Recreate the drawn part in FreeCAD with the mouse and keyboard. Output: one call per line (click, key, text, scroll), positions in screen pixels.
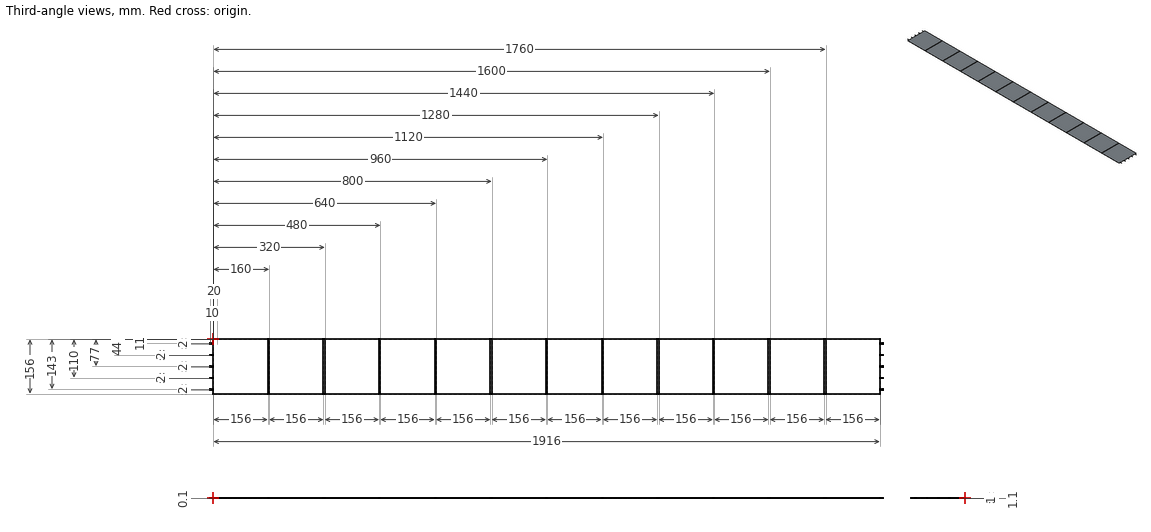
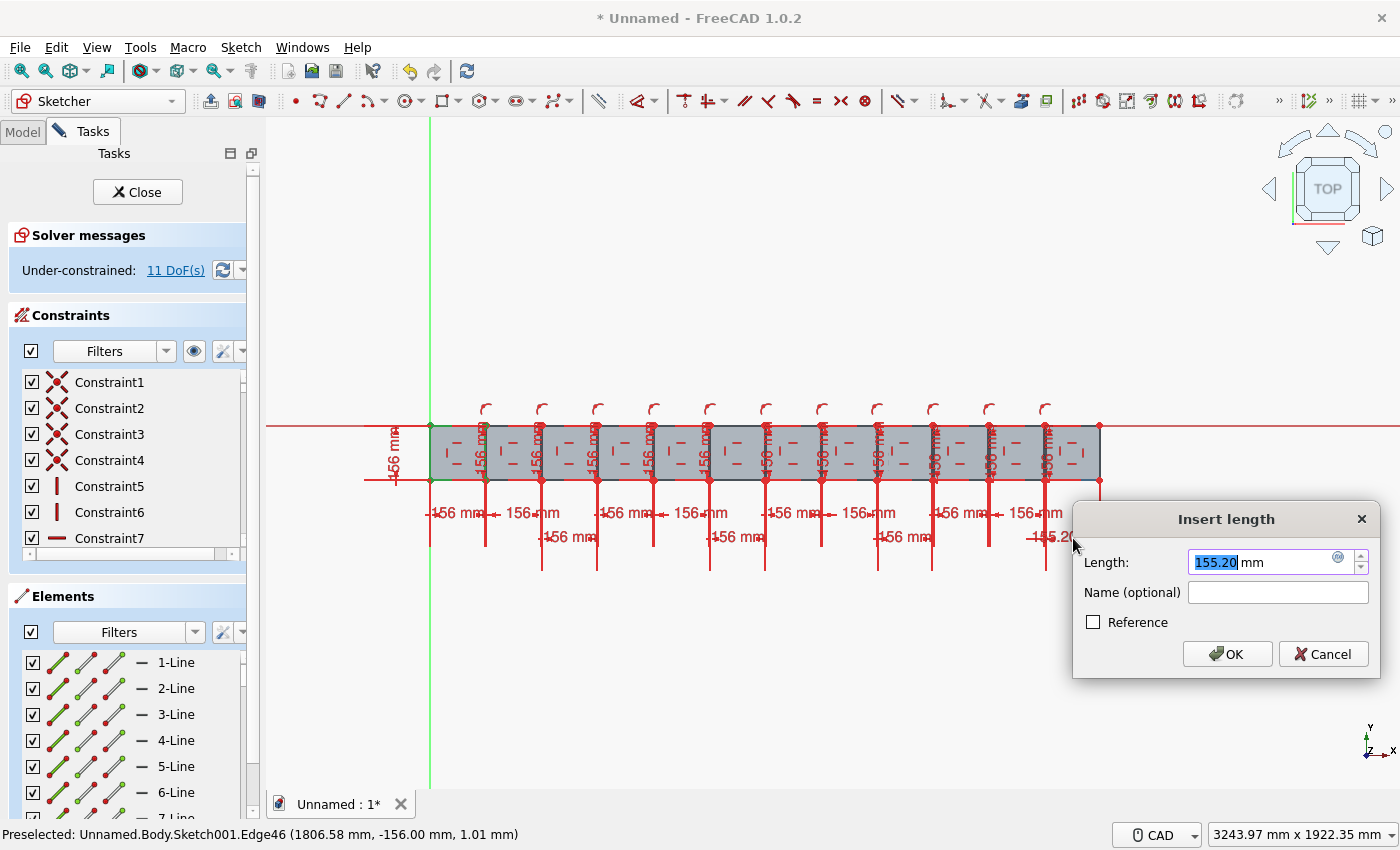
text(156)
key(Return)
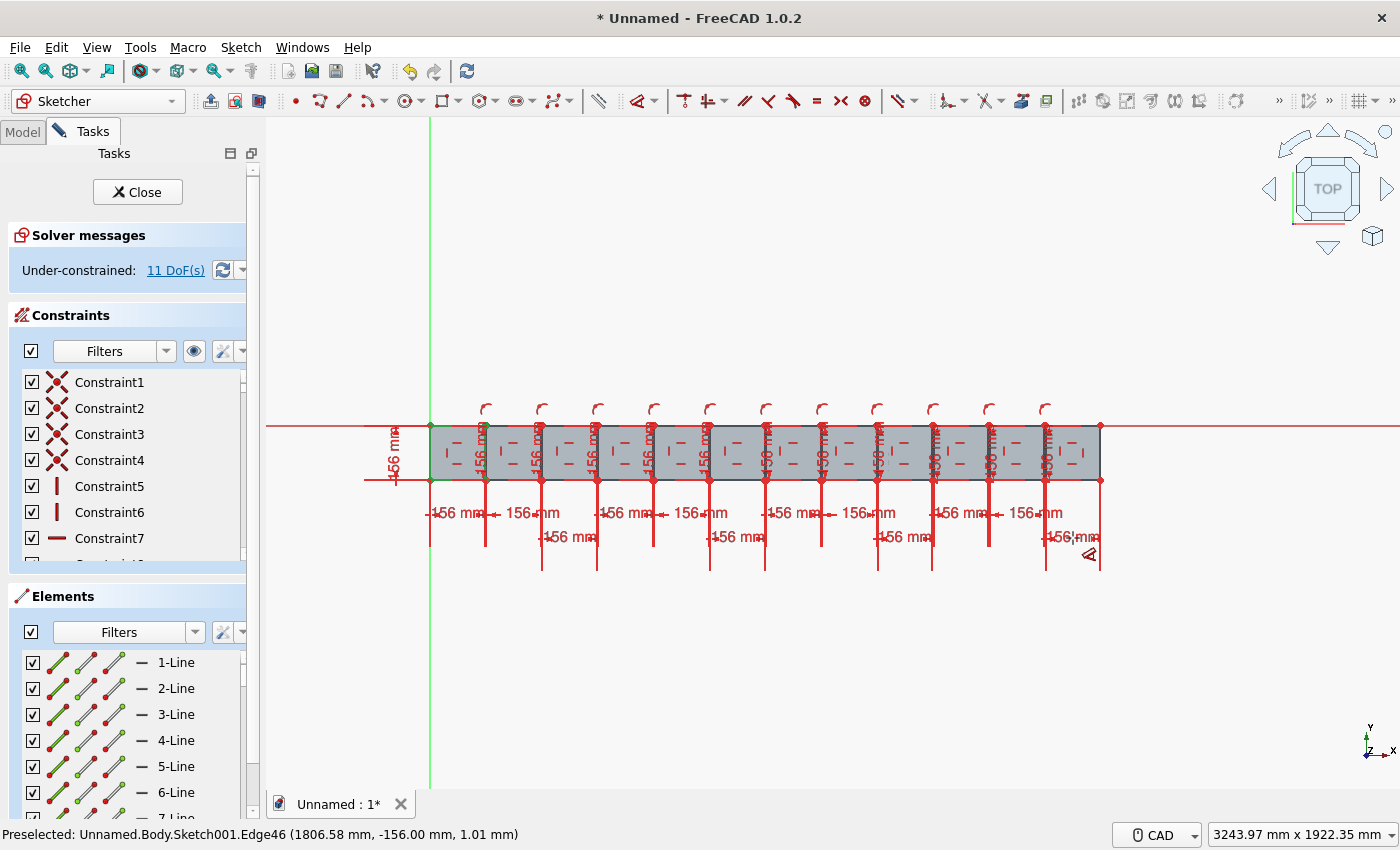
scroll(486, 426, up, 11)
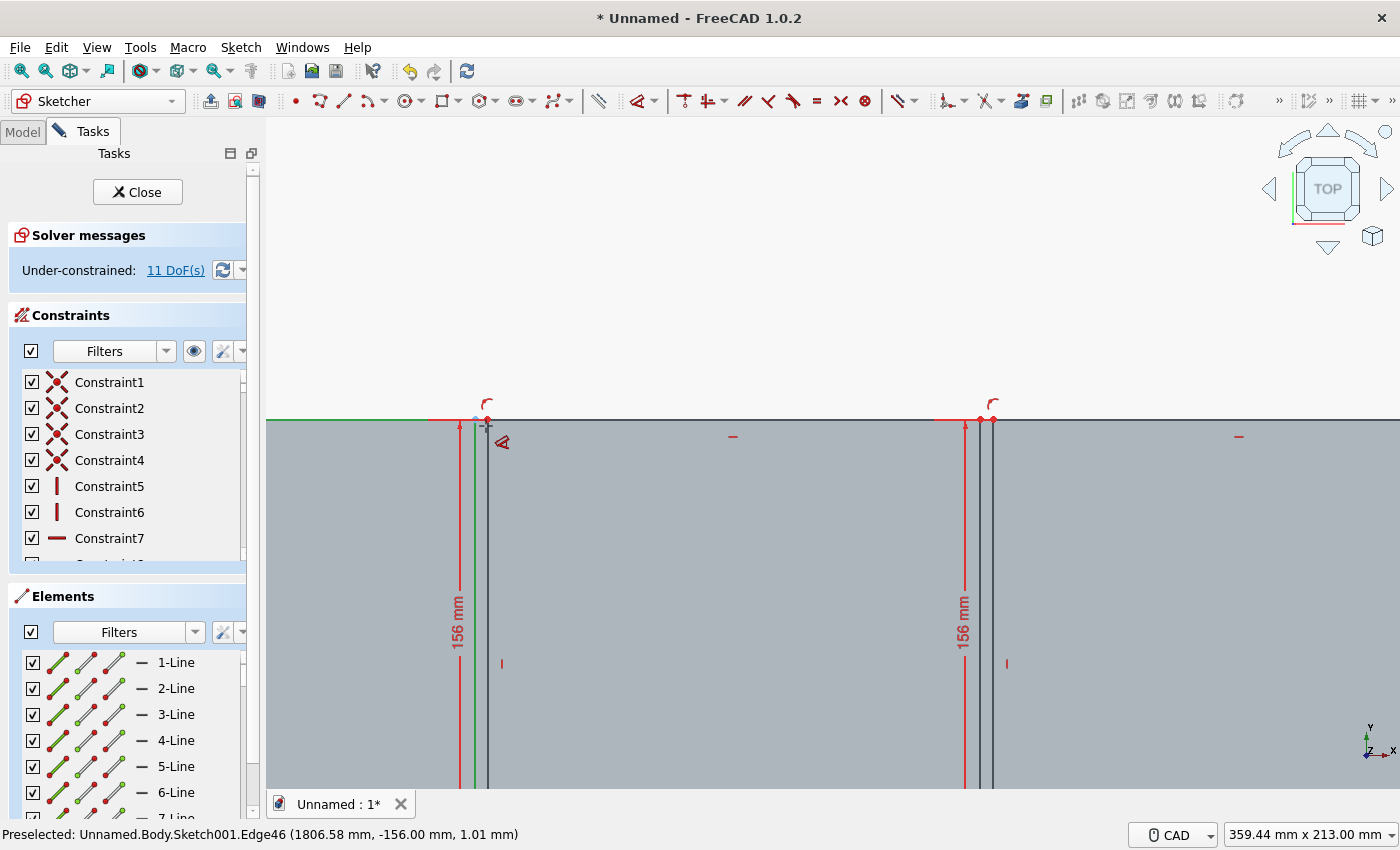
click(488, 420)
click(391, 386)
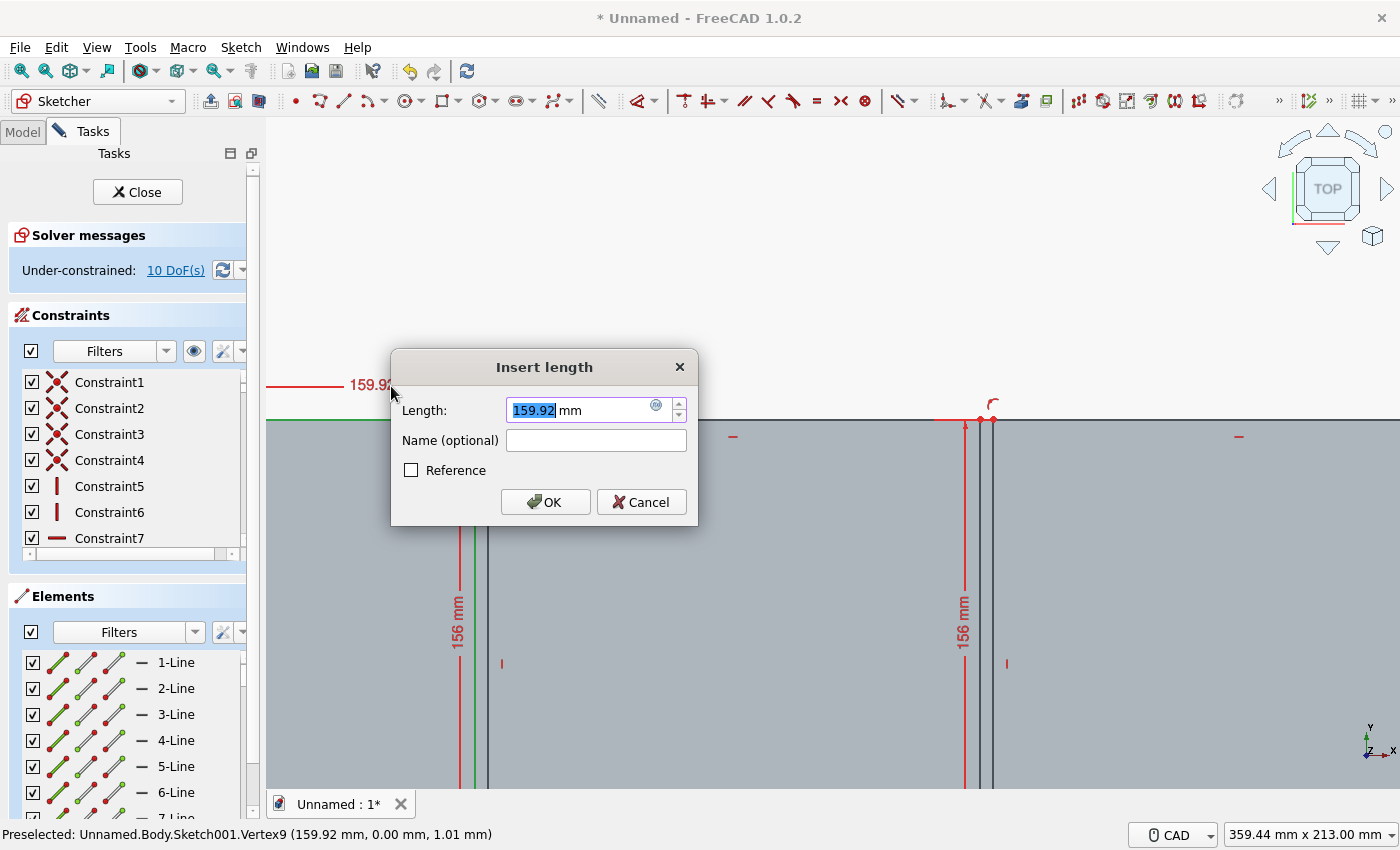
text(160)
key(Return)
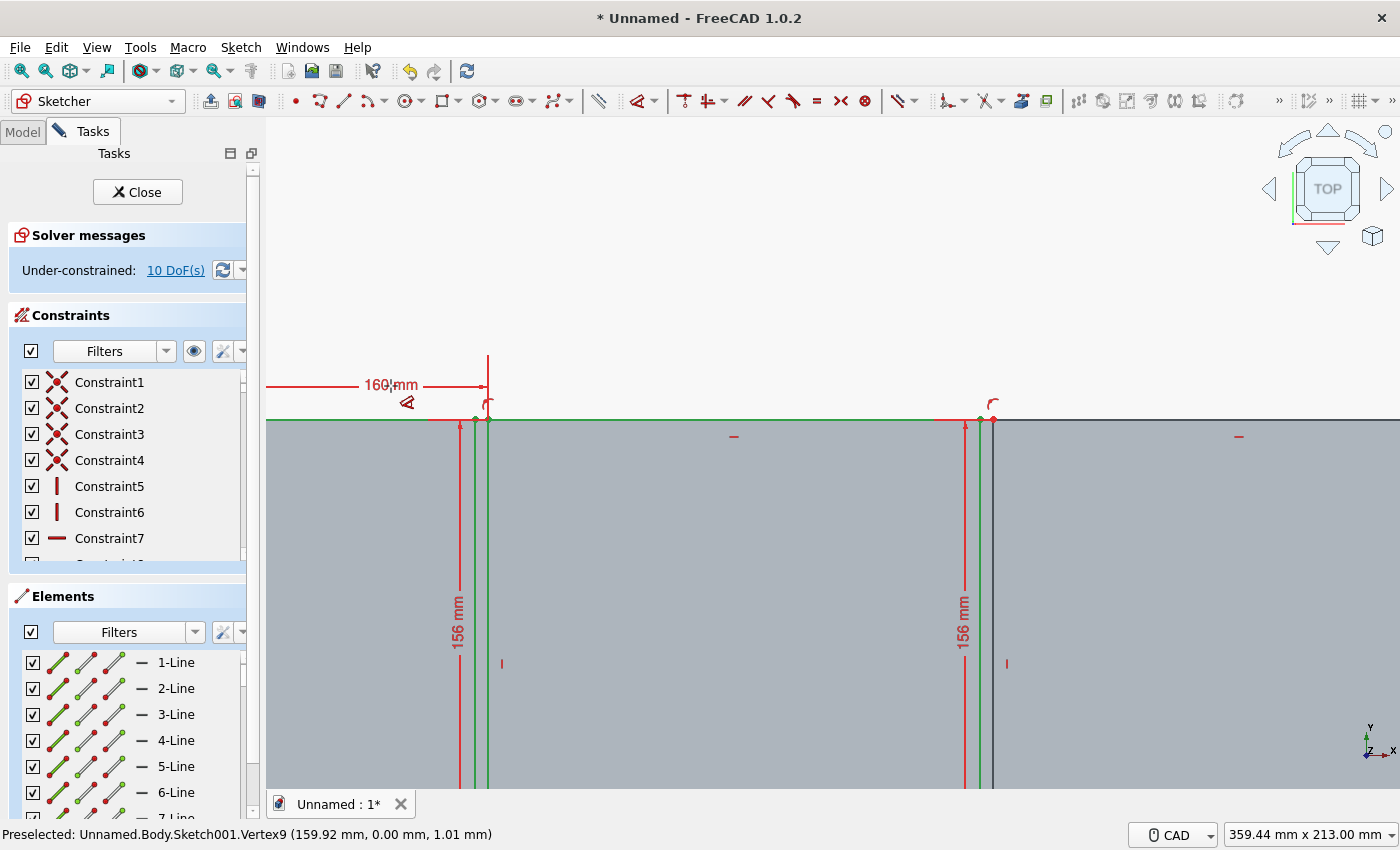
click(993, 420)
click(644, 386)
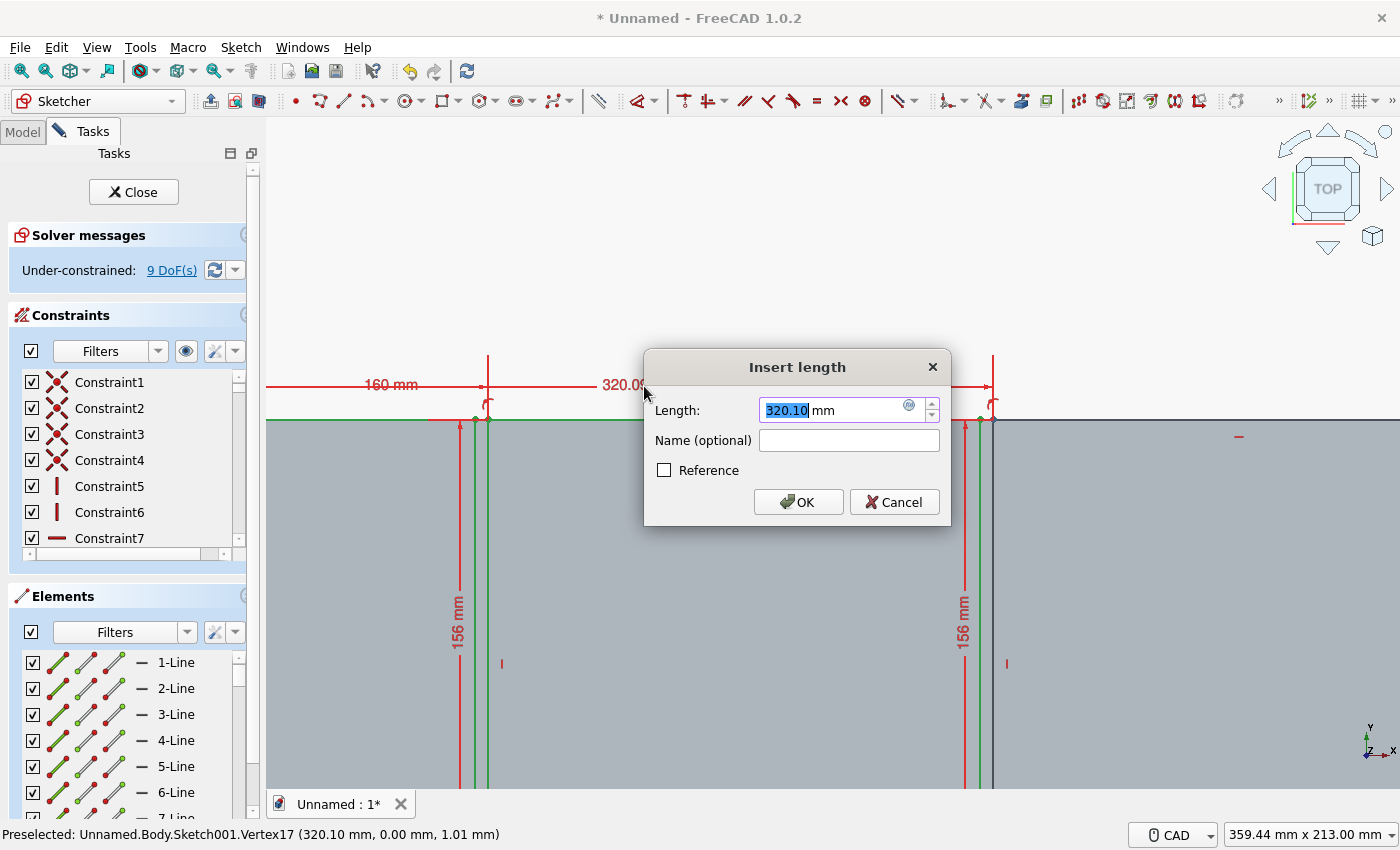
text(320)
key(Return)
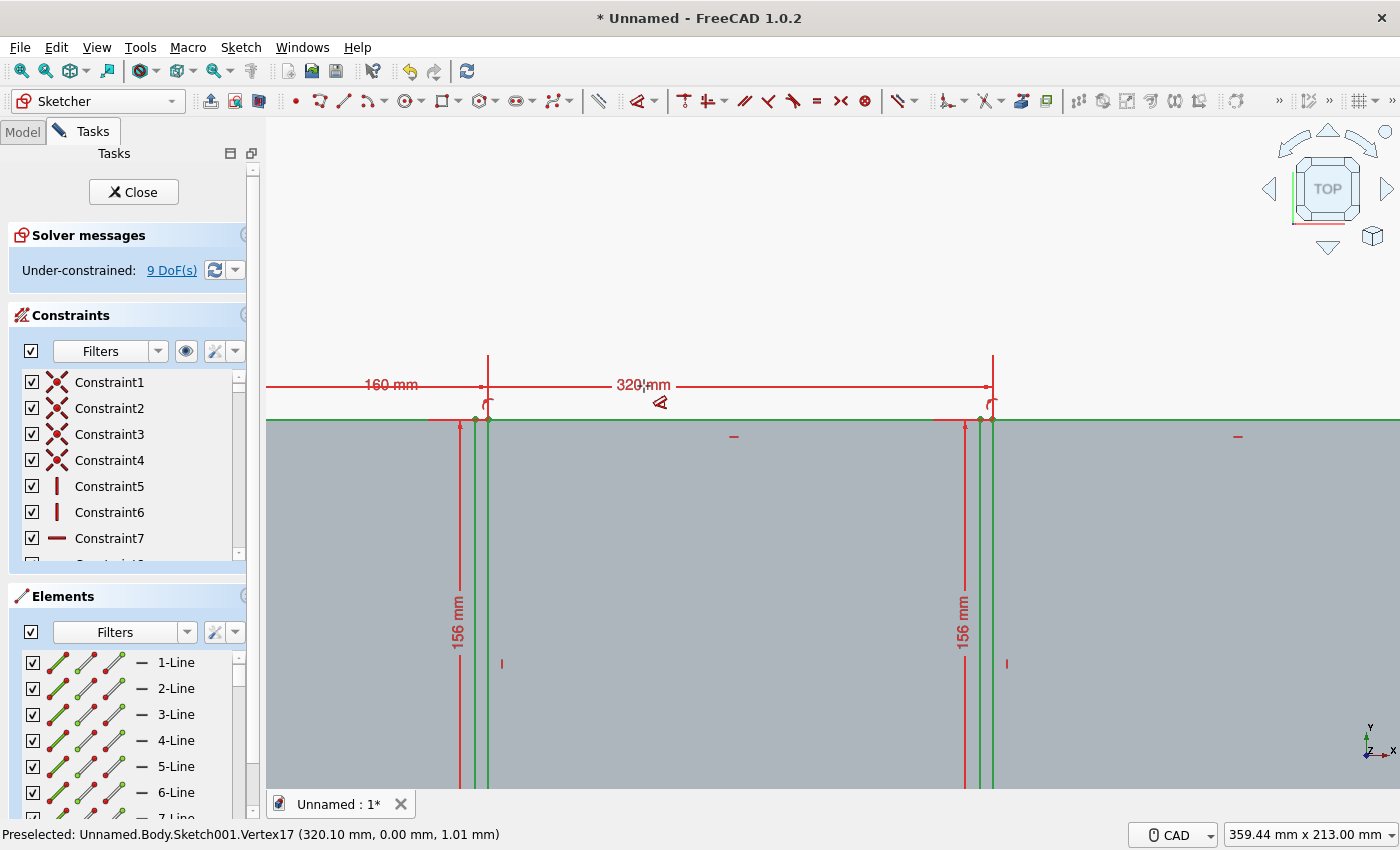
scroll(485, 426, down, 11)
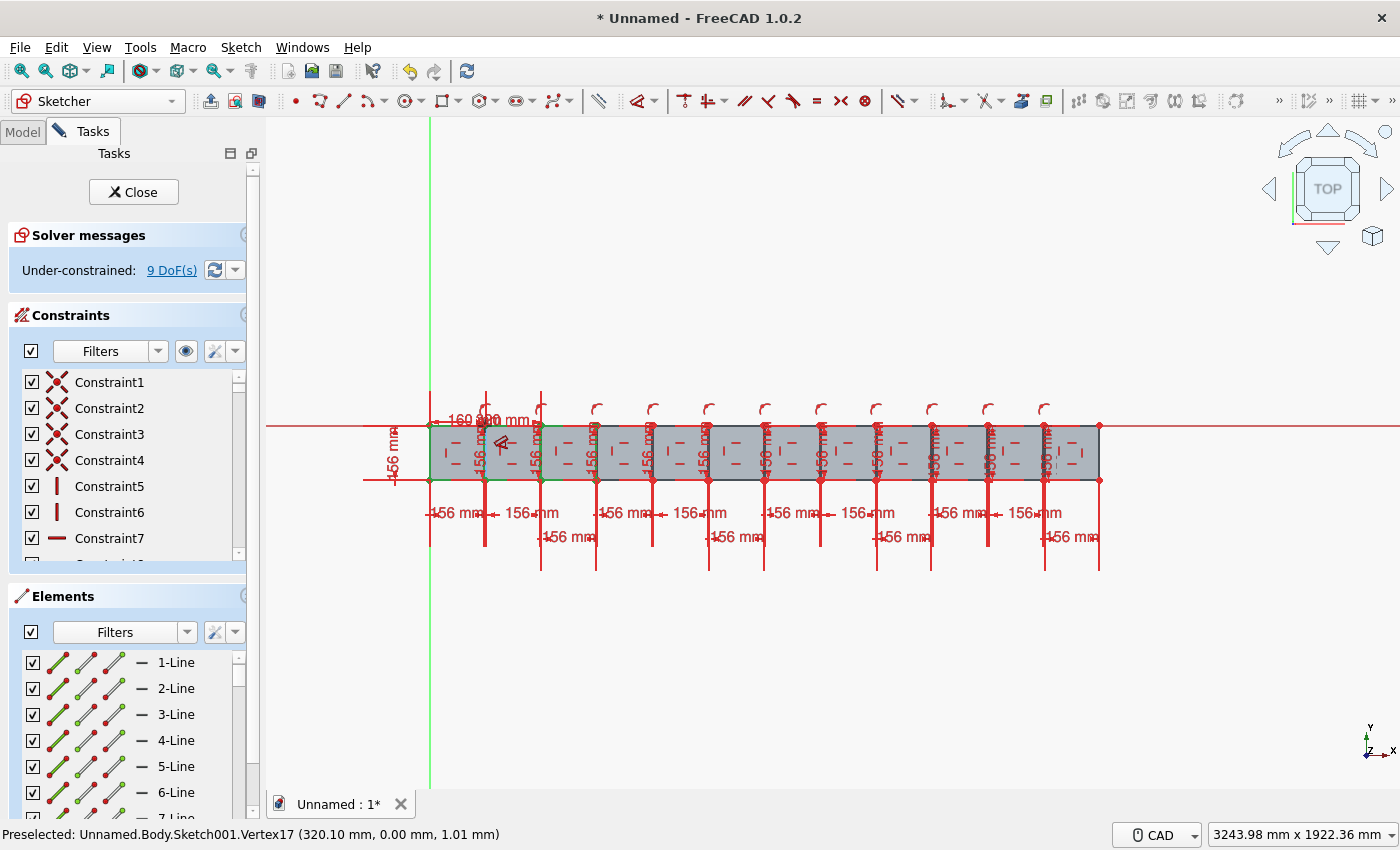
scroll(597, 426, up, 11)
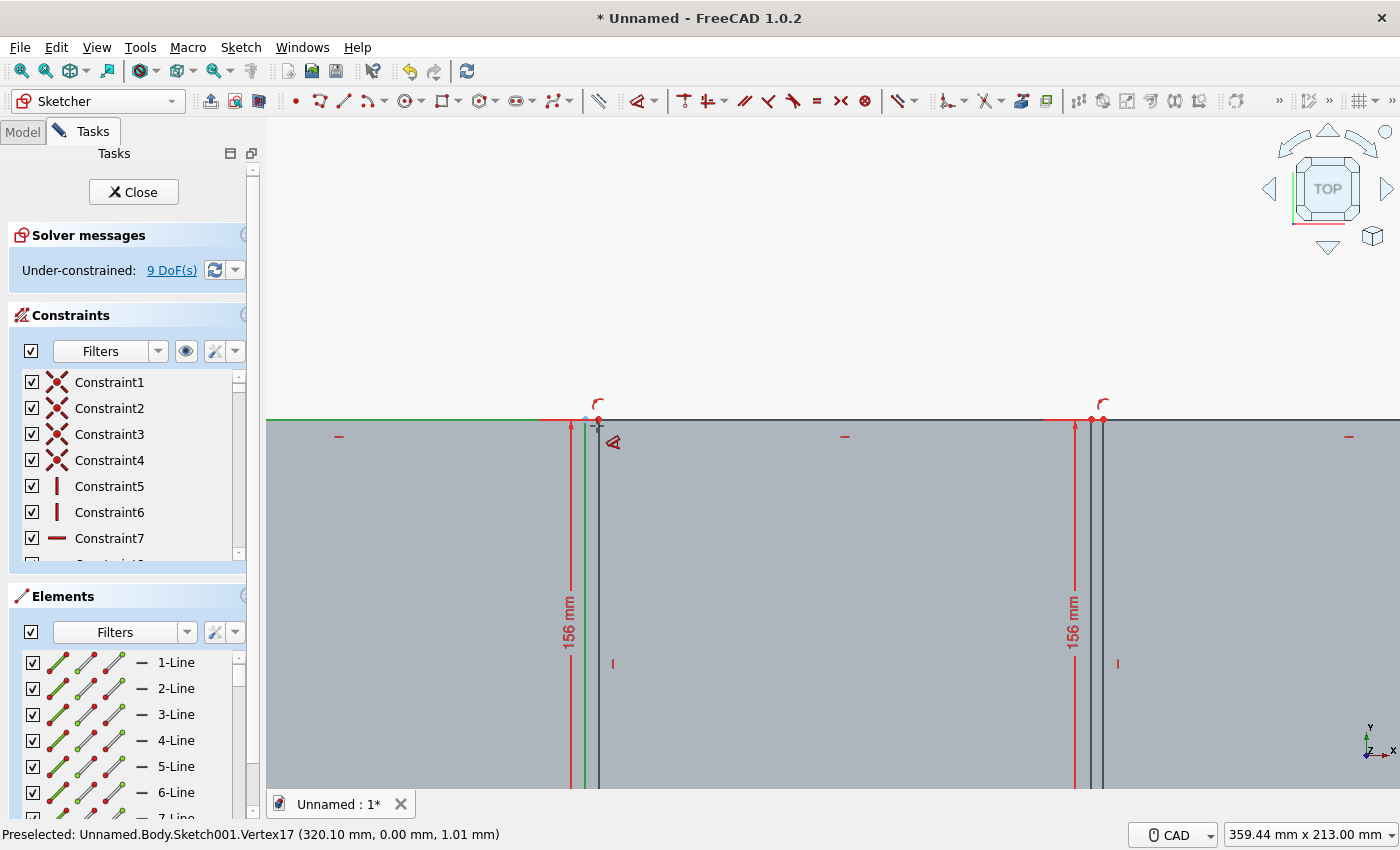
click(599, 420)
click(446, 386)